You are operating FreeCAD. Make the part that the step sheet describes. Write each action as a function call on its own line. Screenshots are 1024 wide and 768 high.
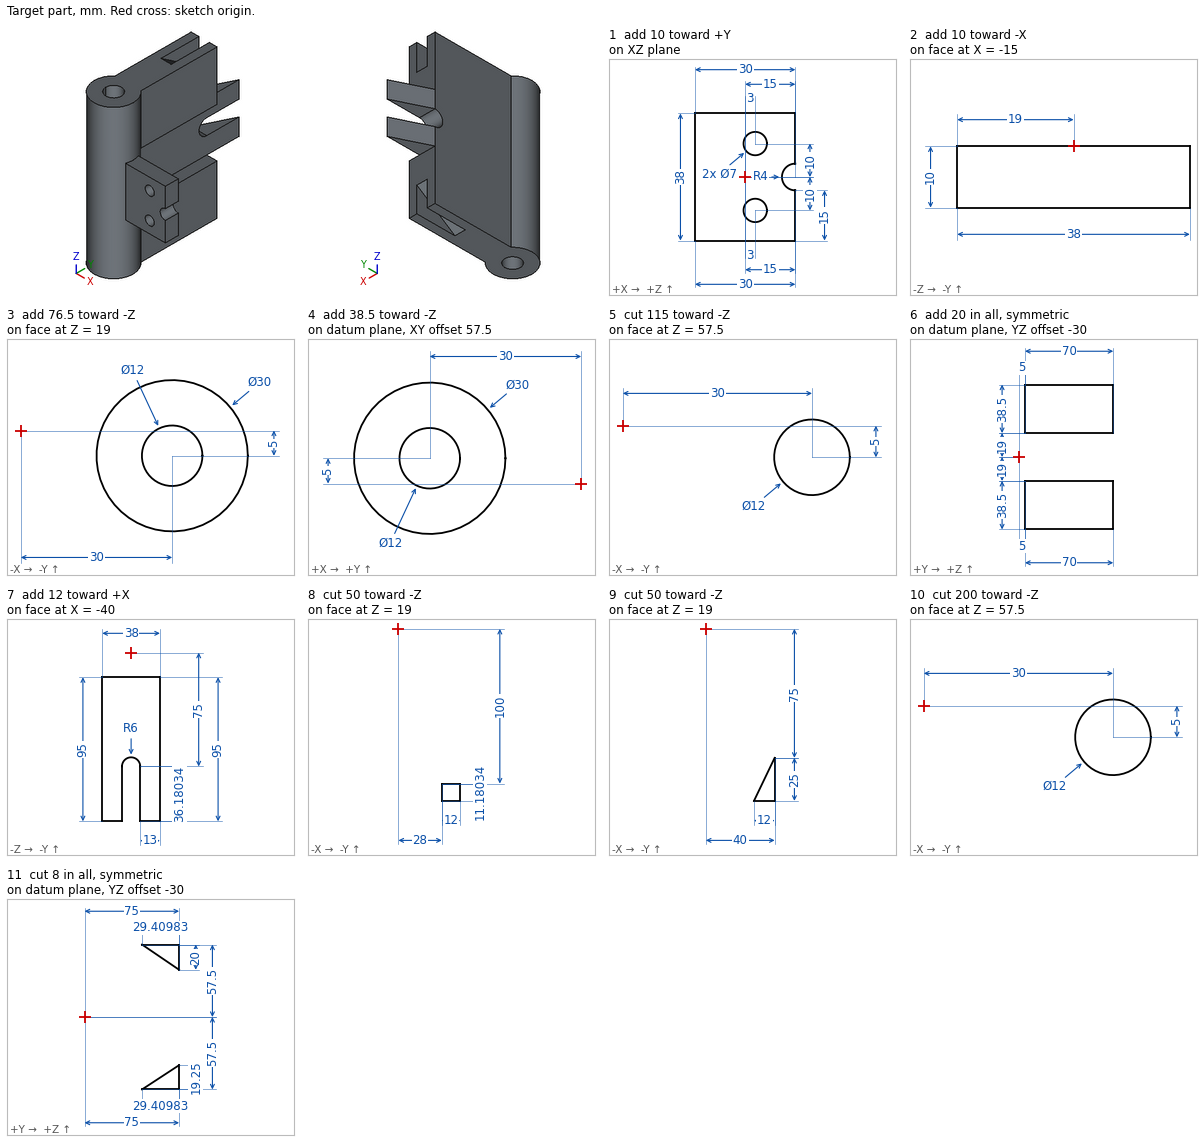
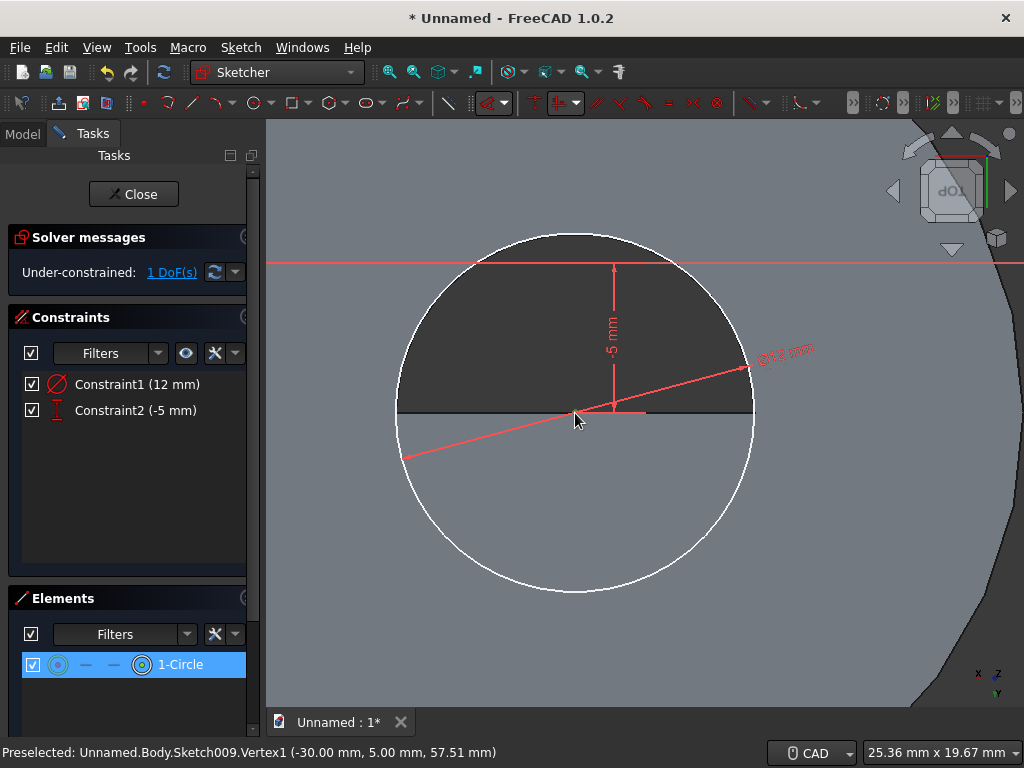
click(506, 104)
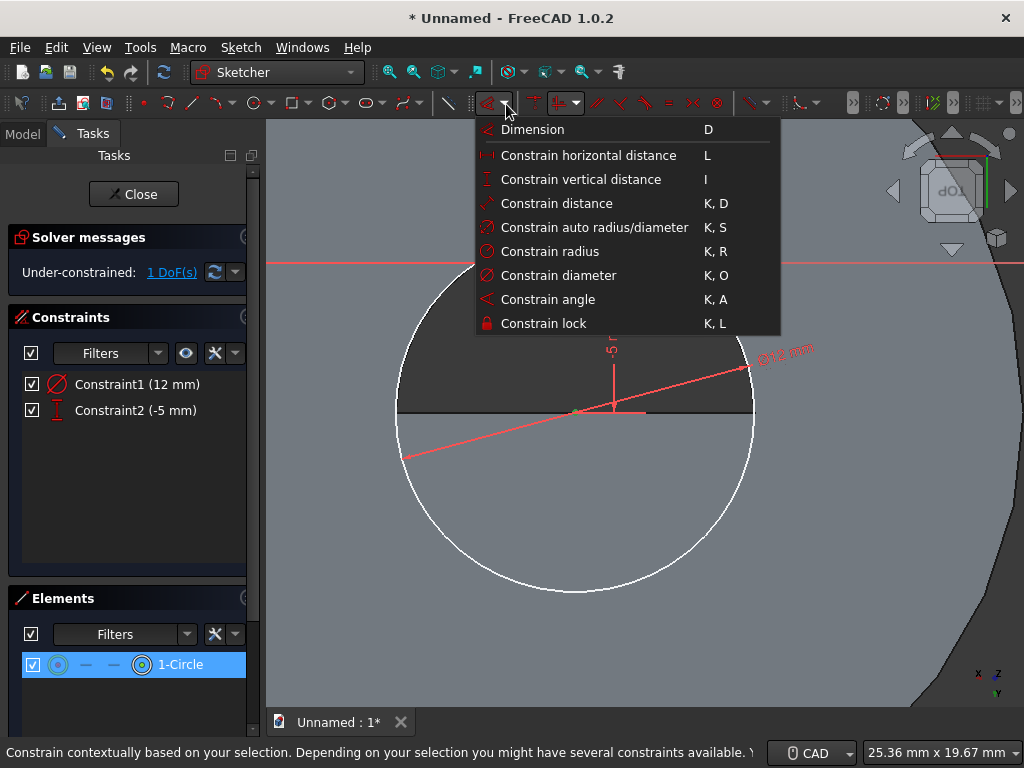
click(628, 155)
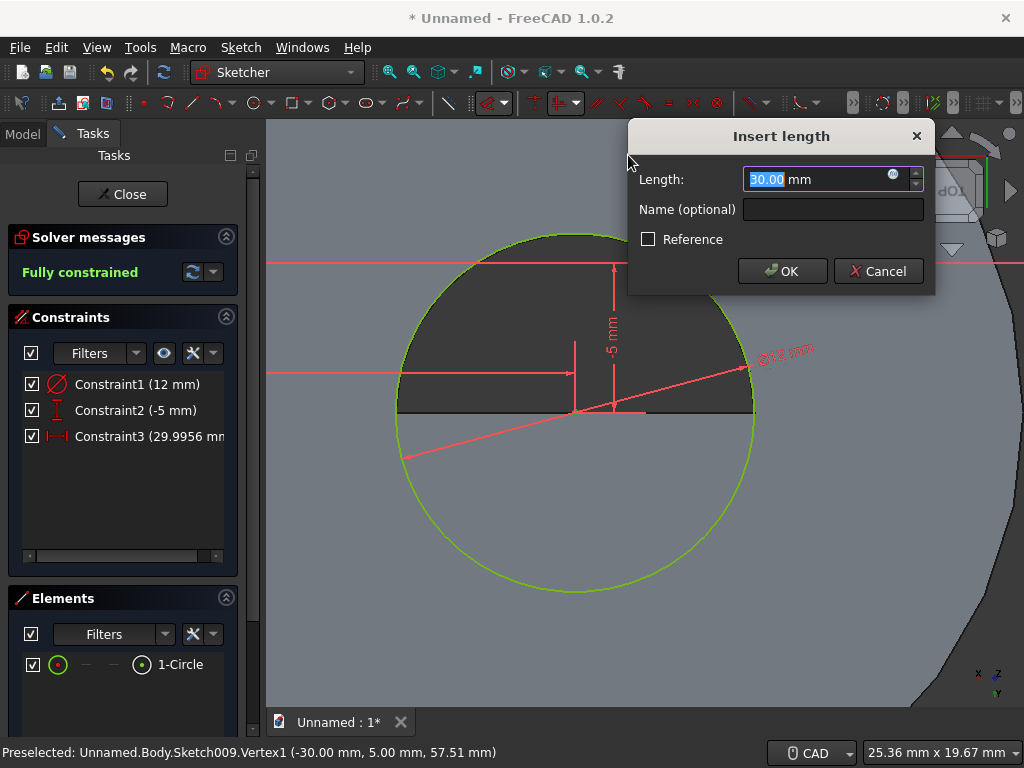
text(30)
key(Return)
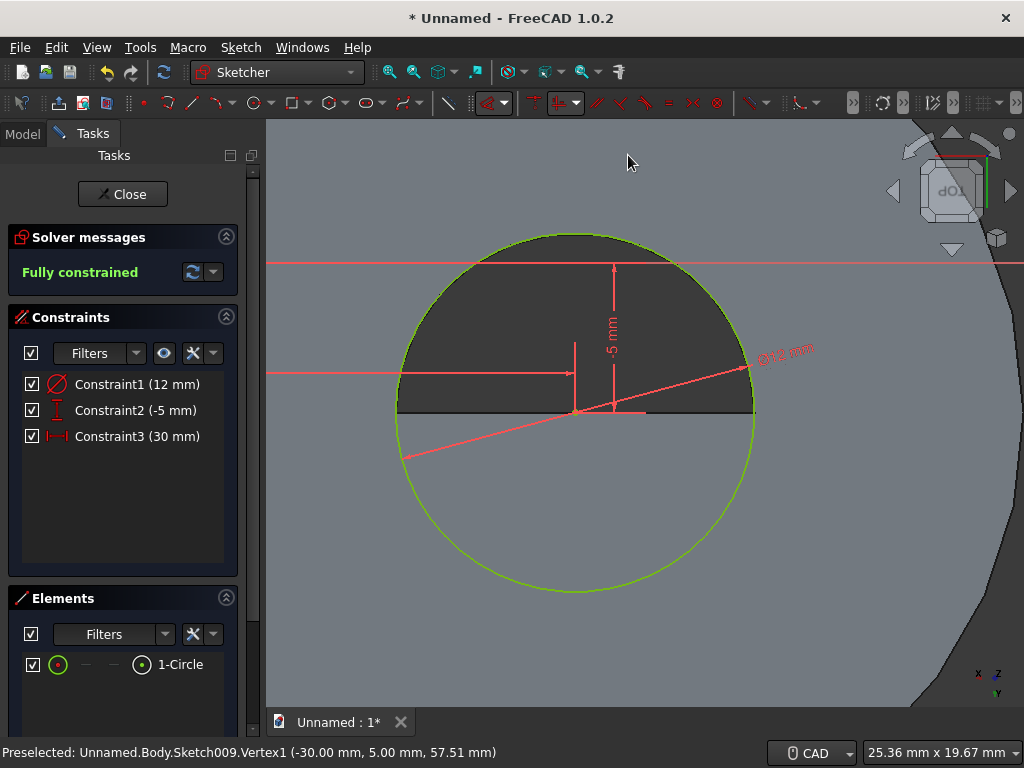
click(123, 194)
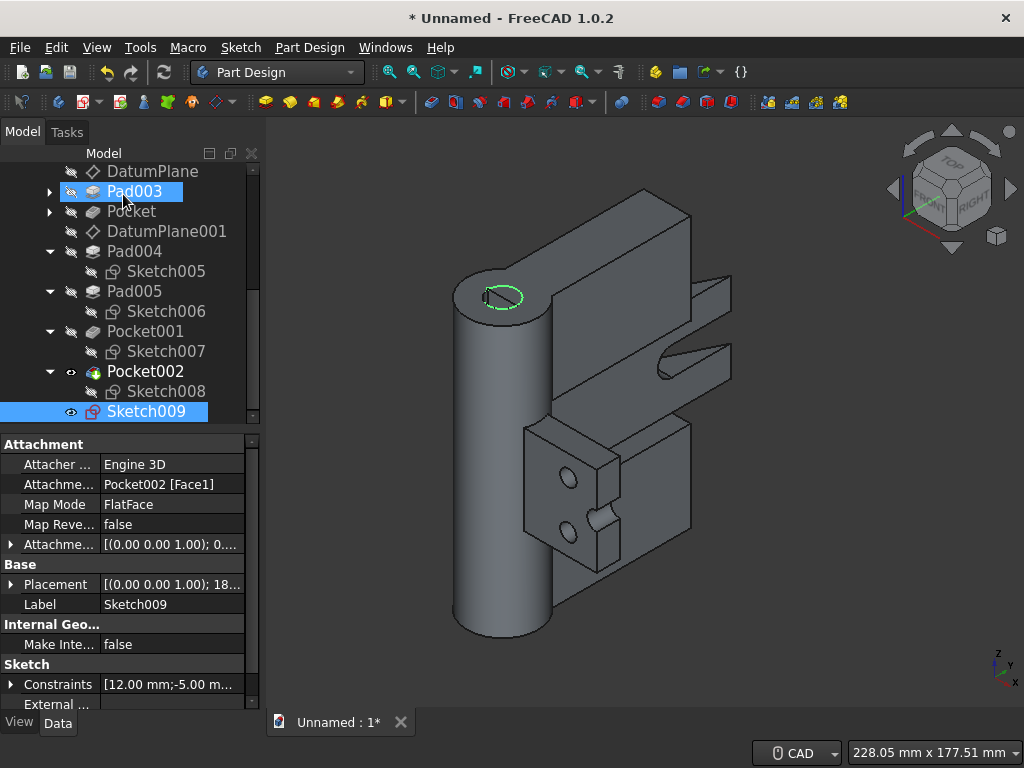
click(432, 102)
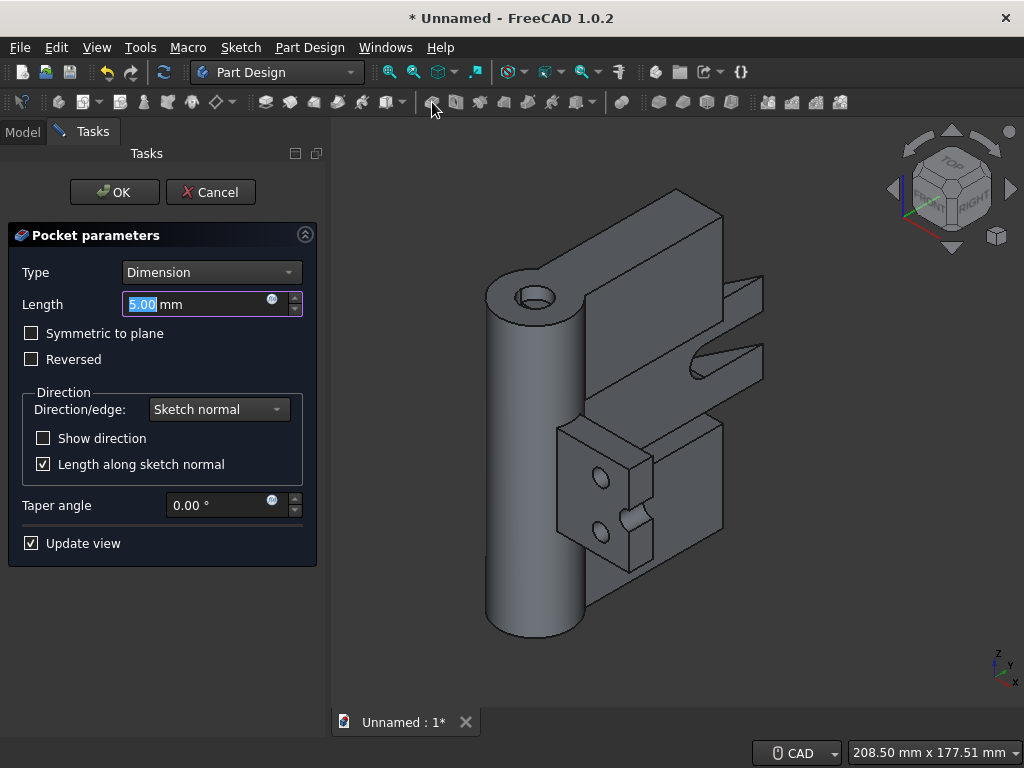
text(200)
key(Tab)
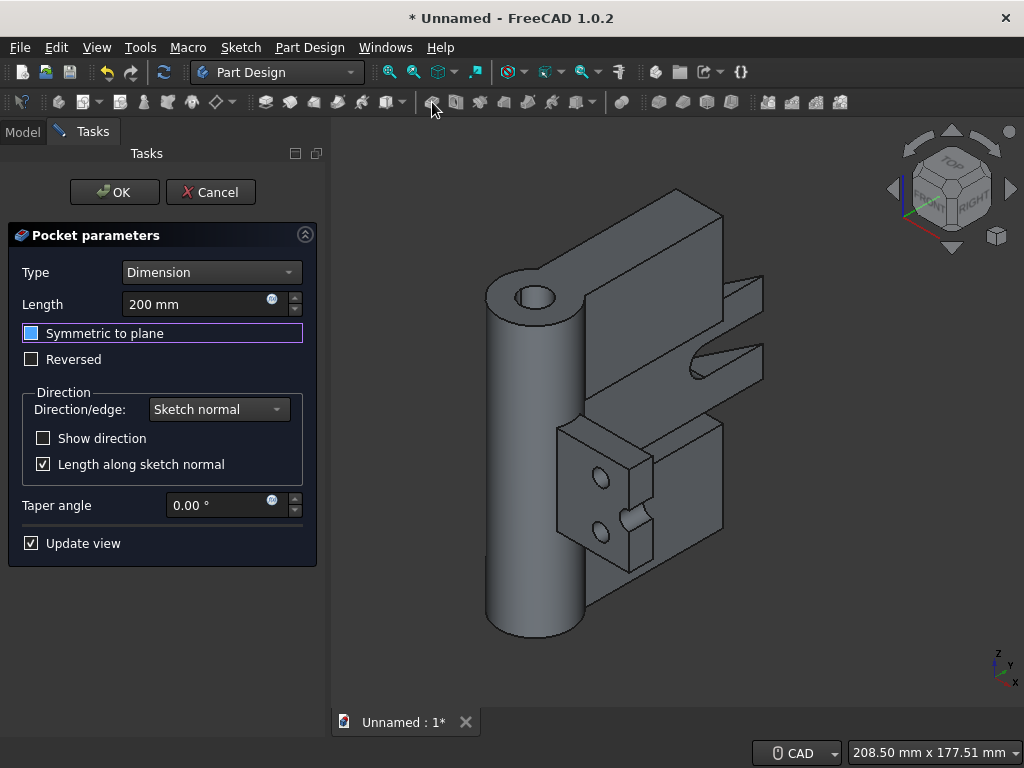
click(115, 192)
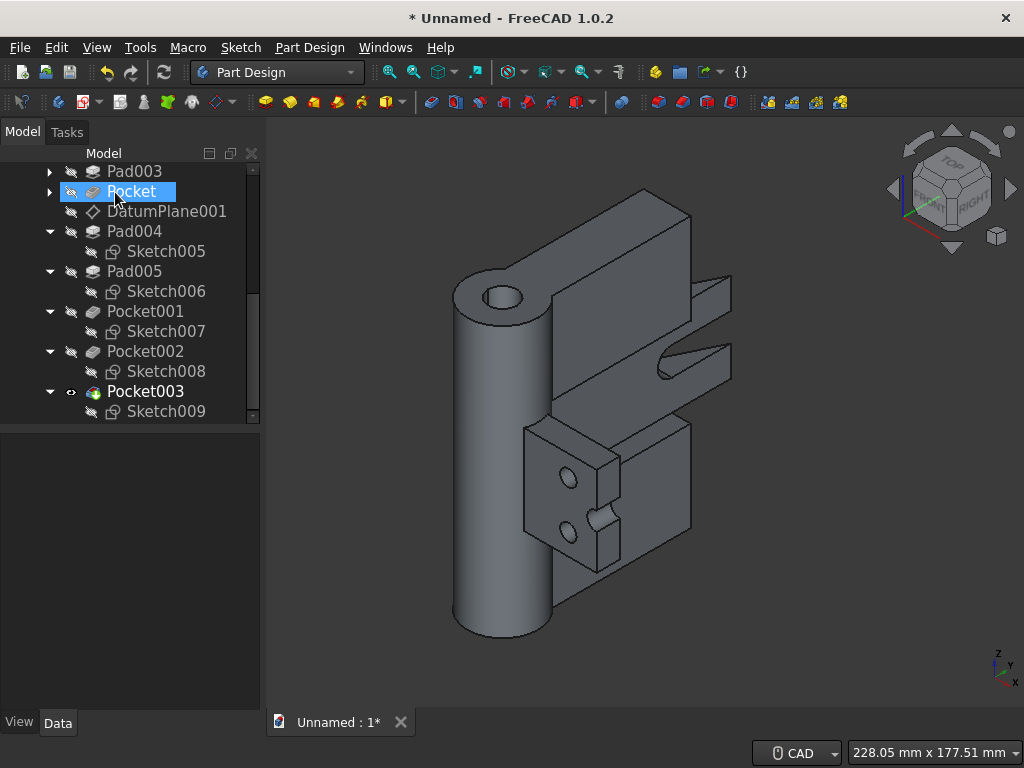
scroll(140, 287, down, 3)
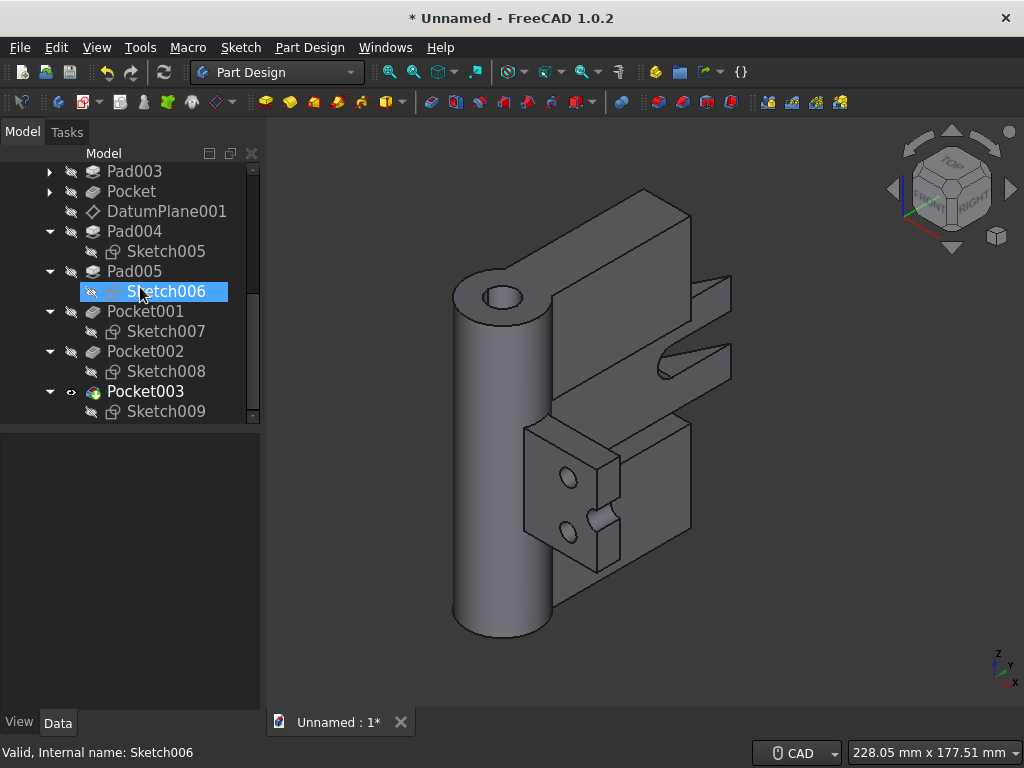
scroll(140, 287, up, 15)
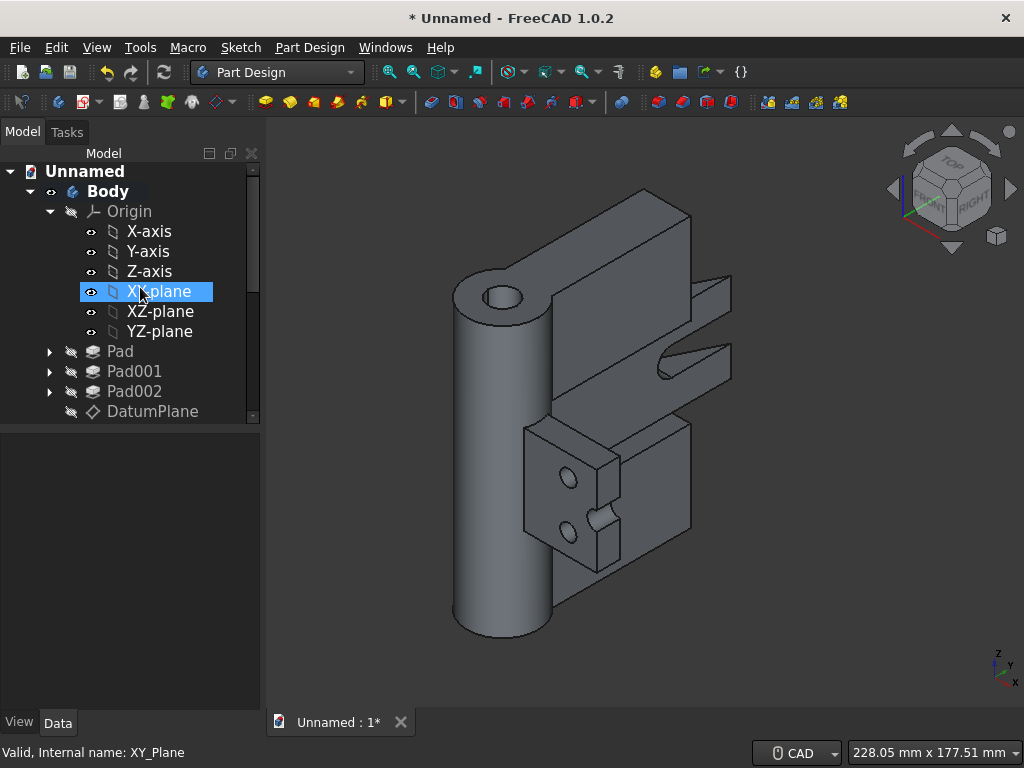
click(136, 332)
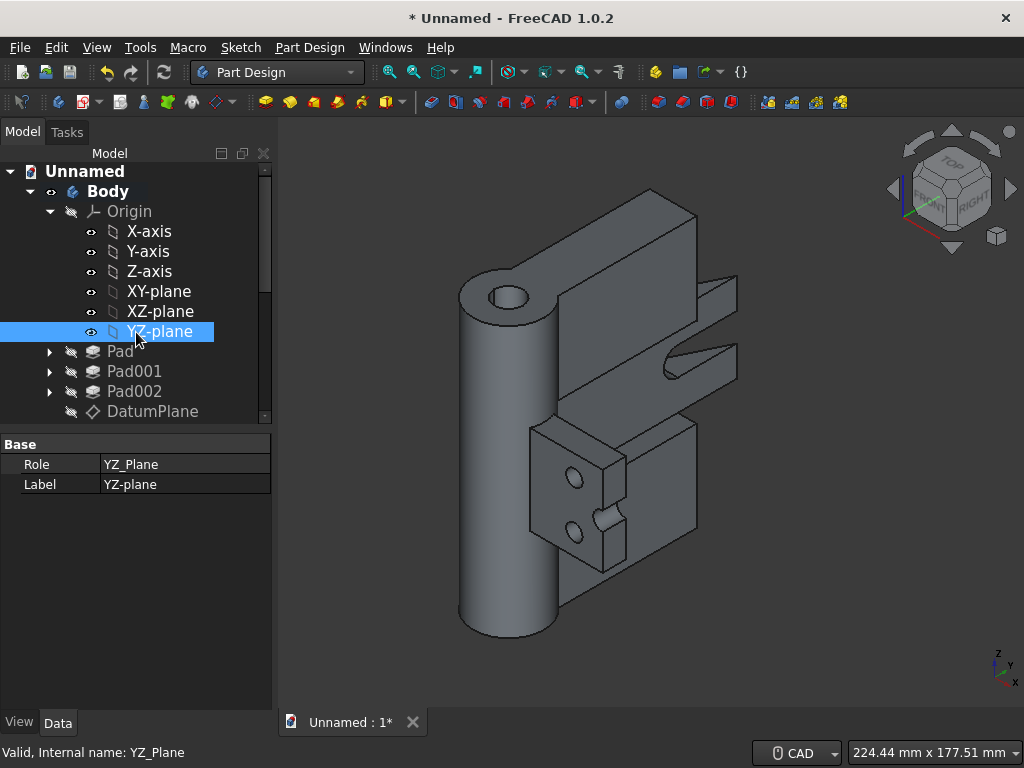
click(216, 102)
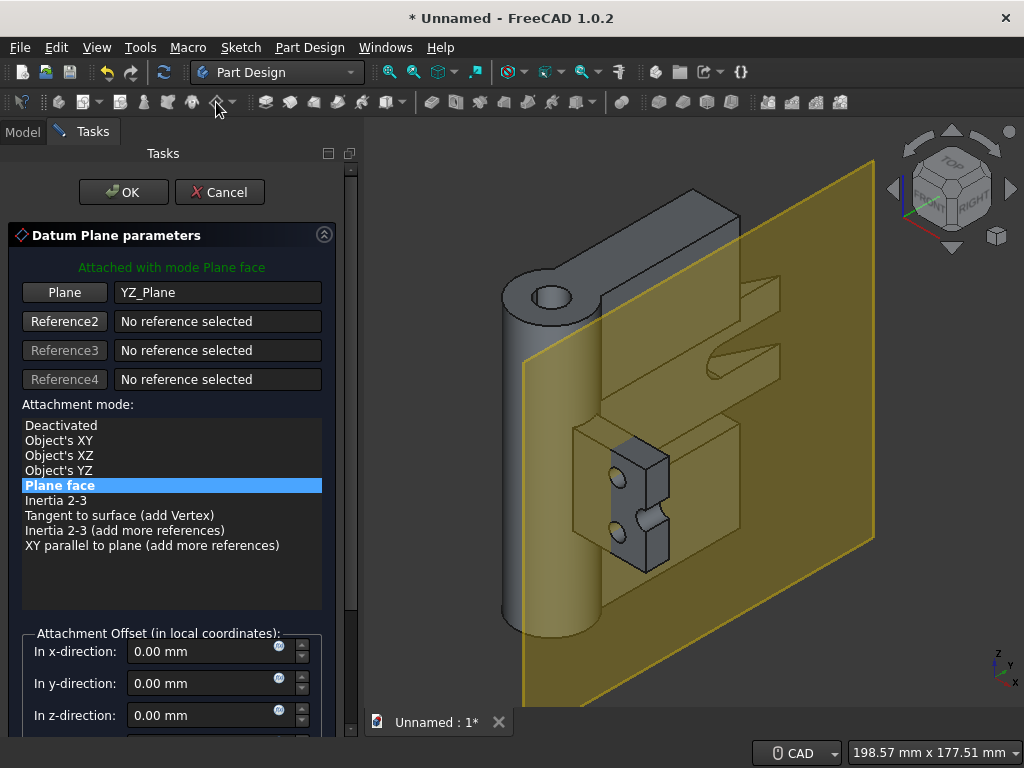
triple_click(210, 715)